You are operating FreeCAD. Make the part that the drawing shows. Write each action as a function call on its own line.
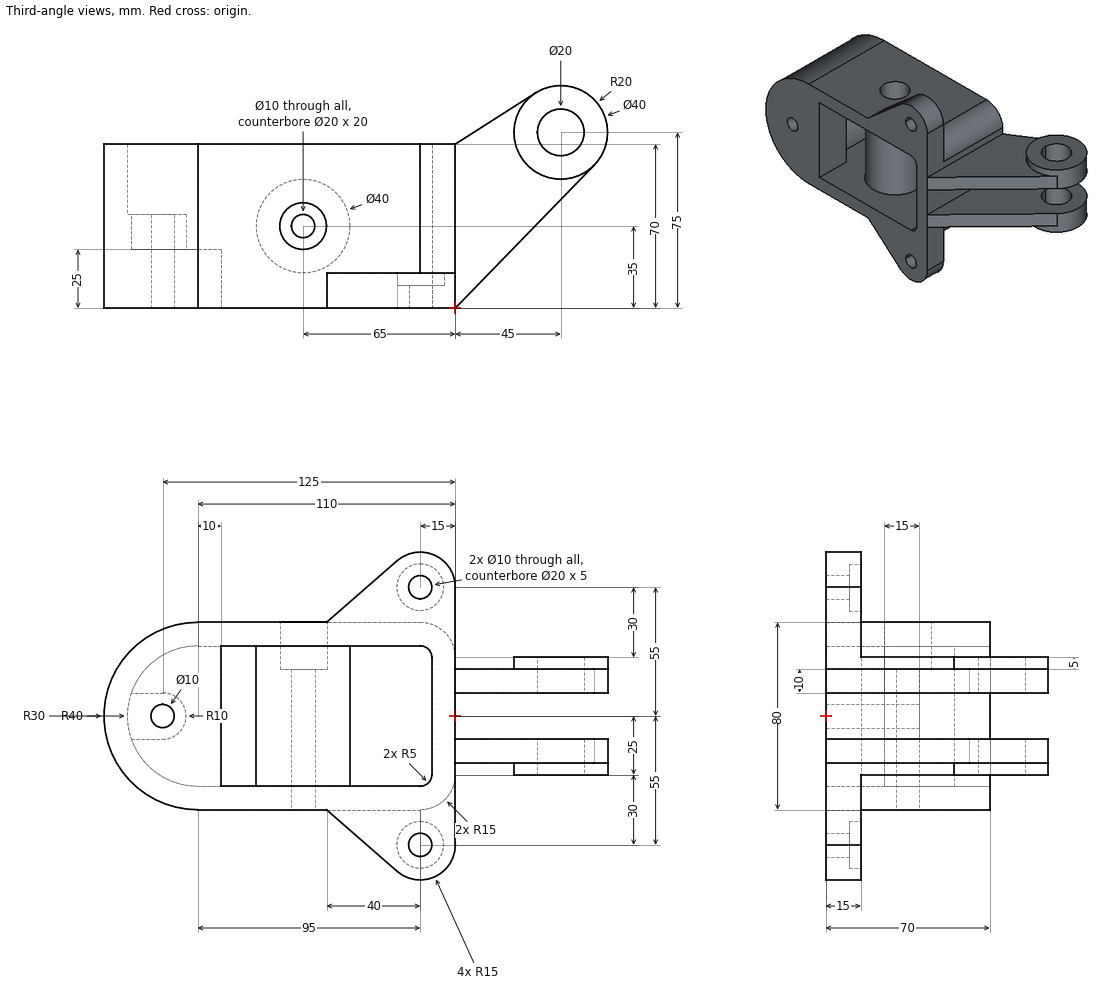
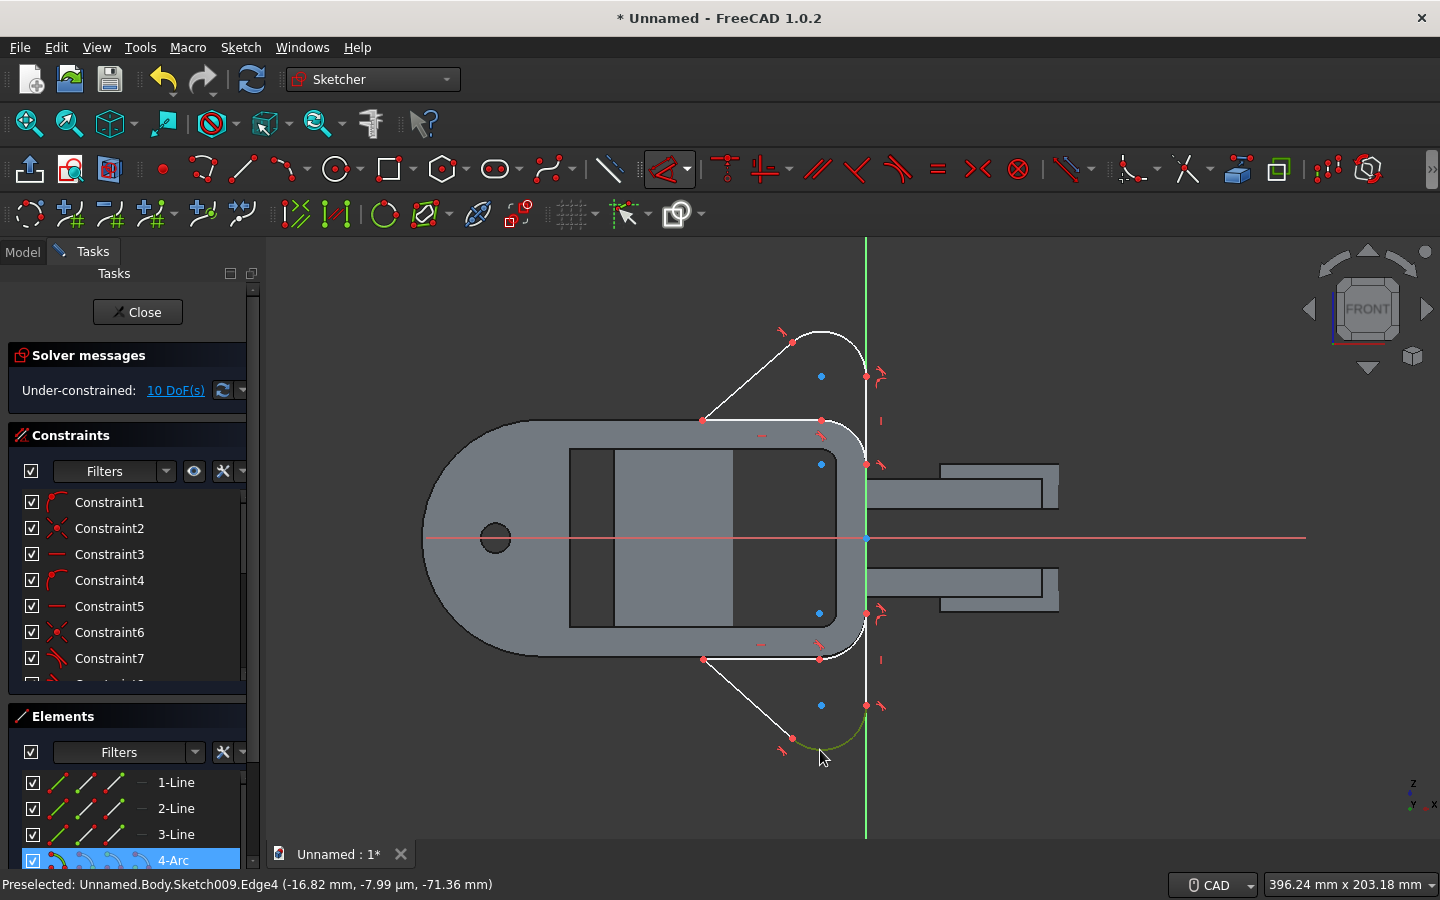
click(841, 654)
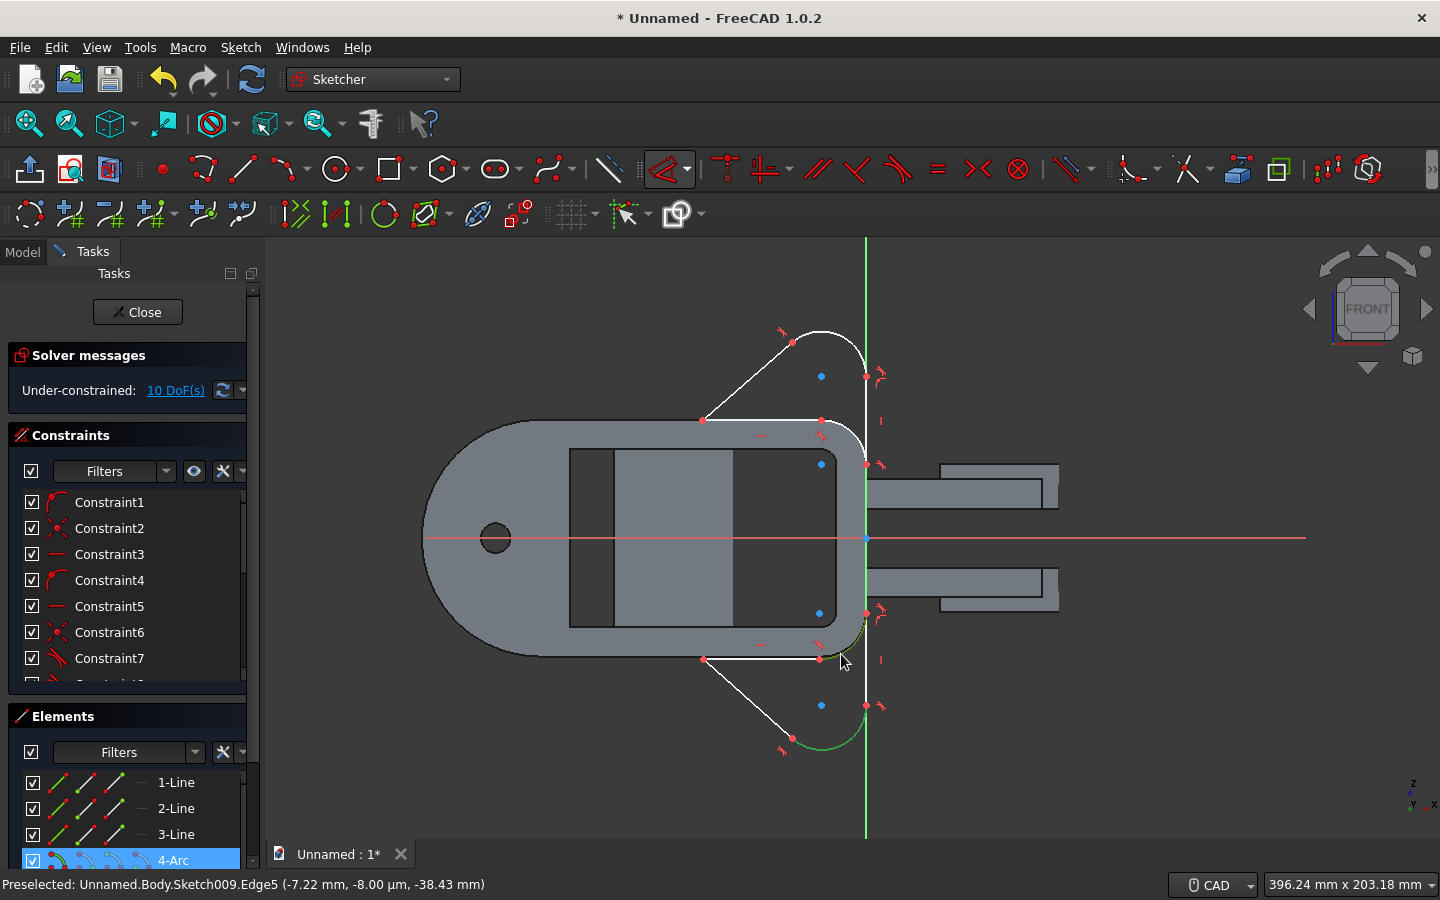
click(842, 425)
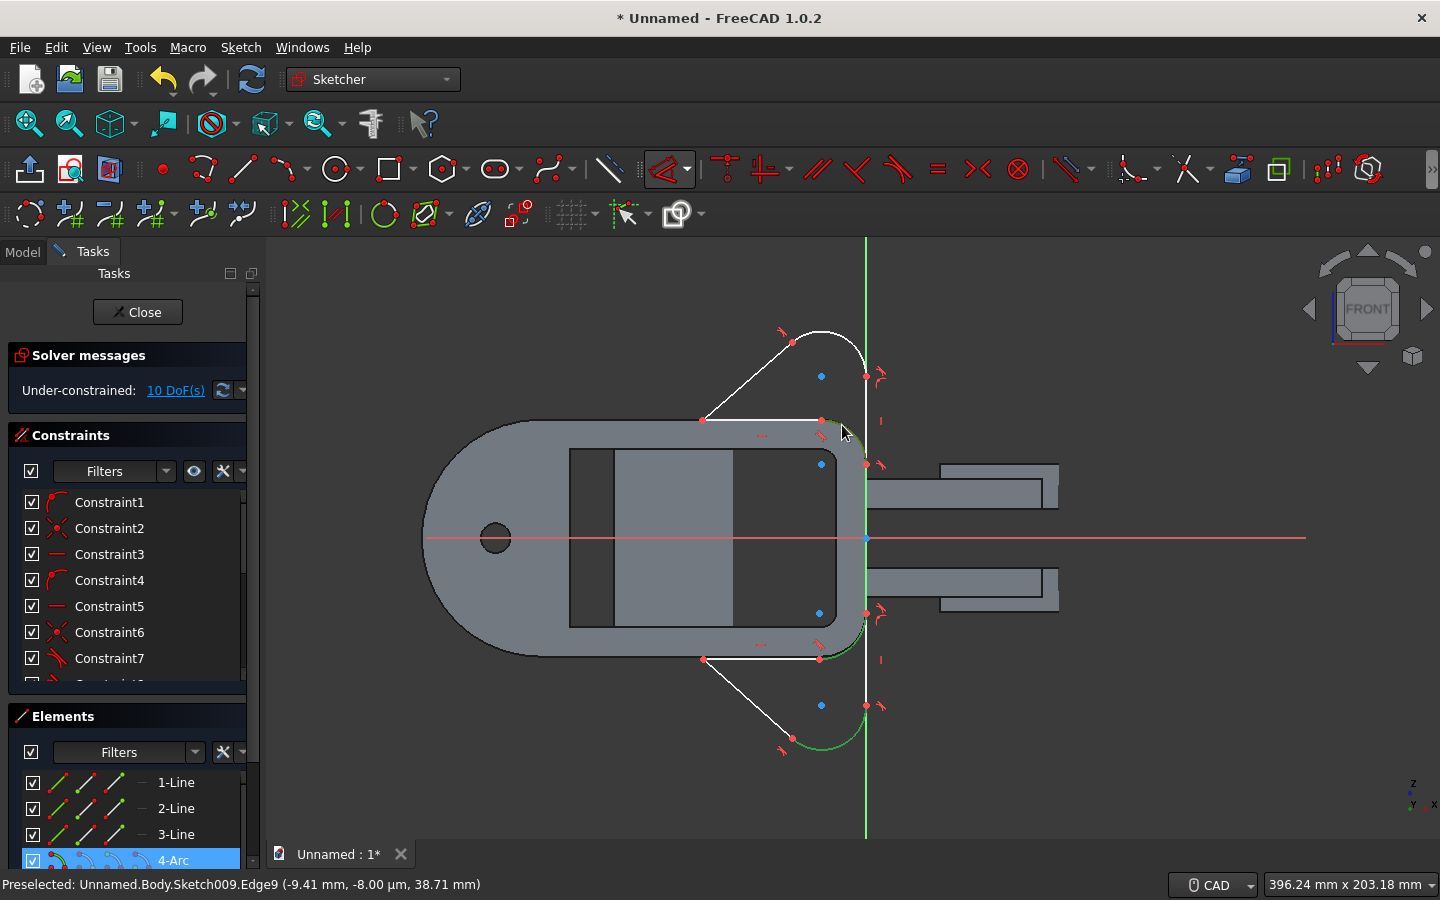
scroll(856, 348, up, 2)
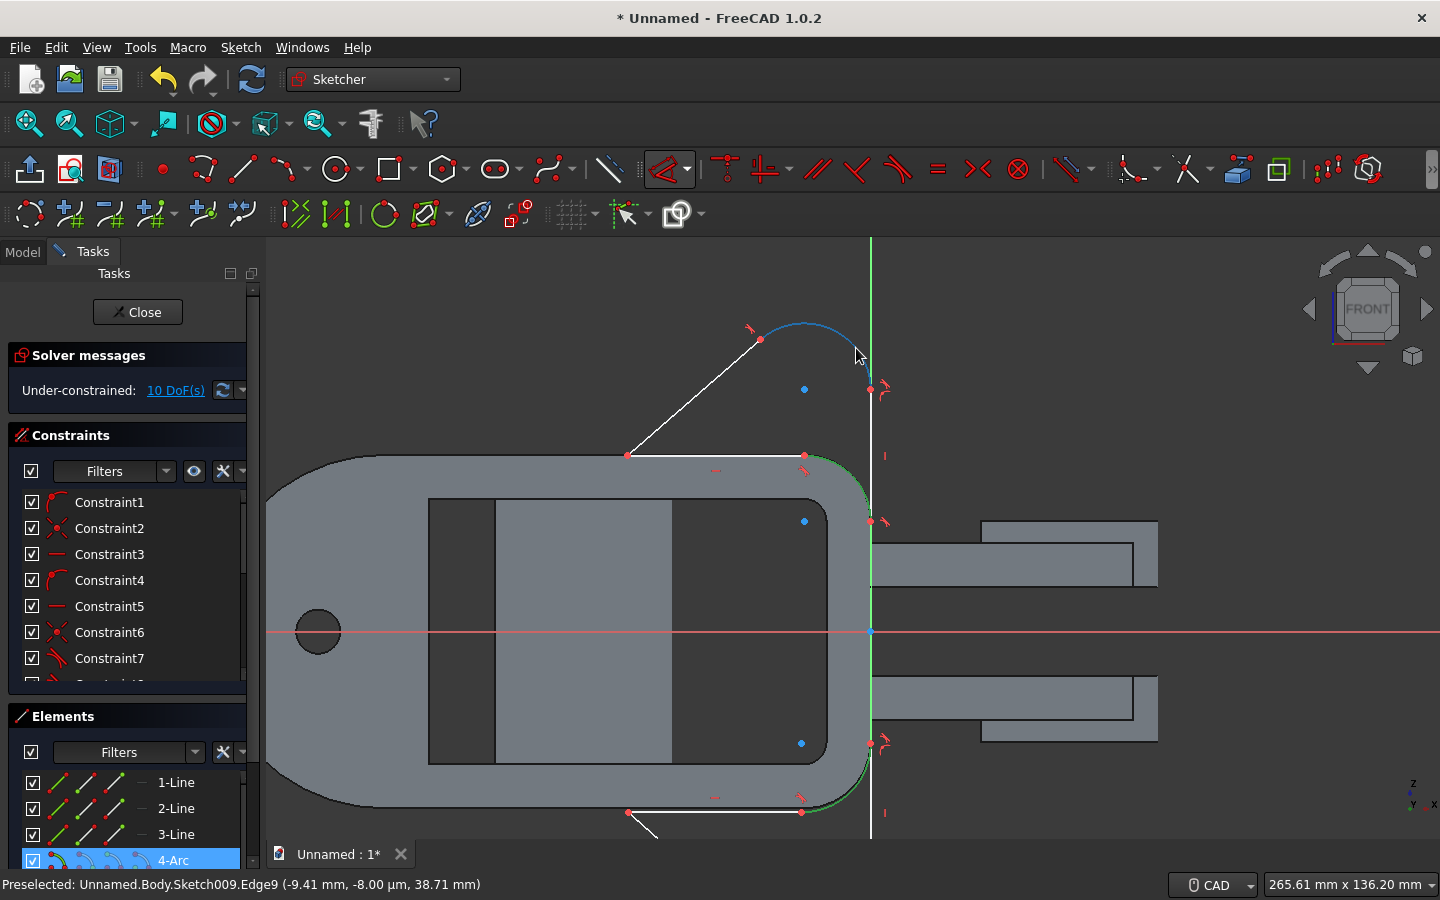
click(856, 348)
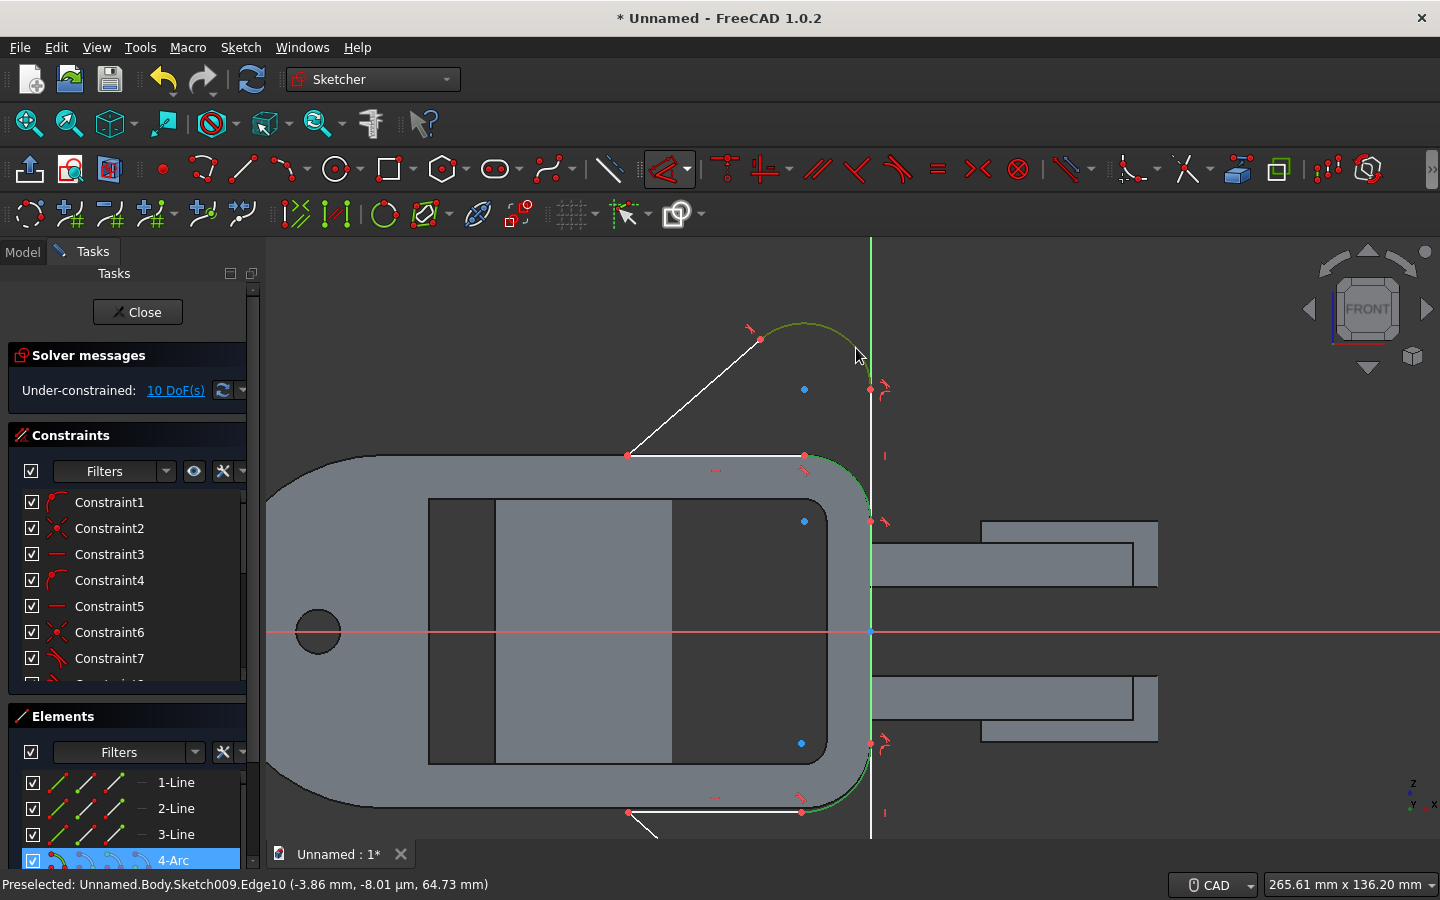
key(e)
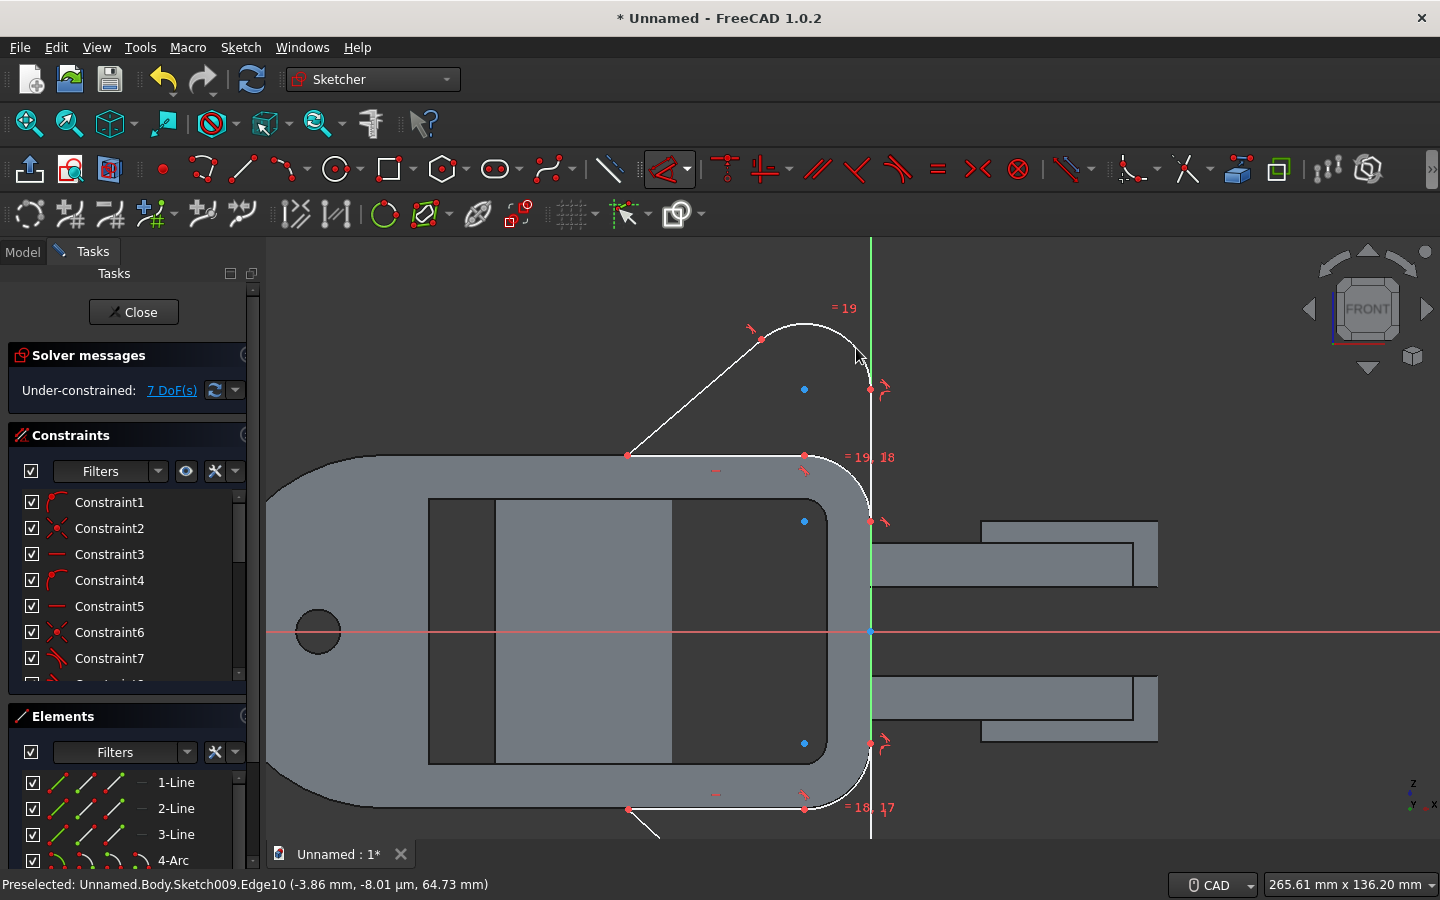
scroll(856, 348, down, 2)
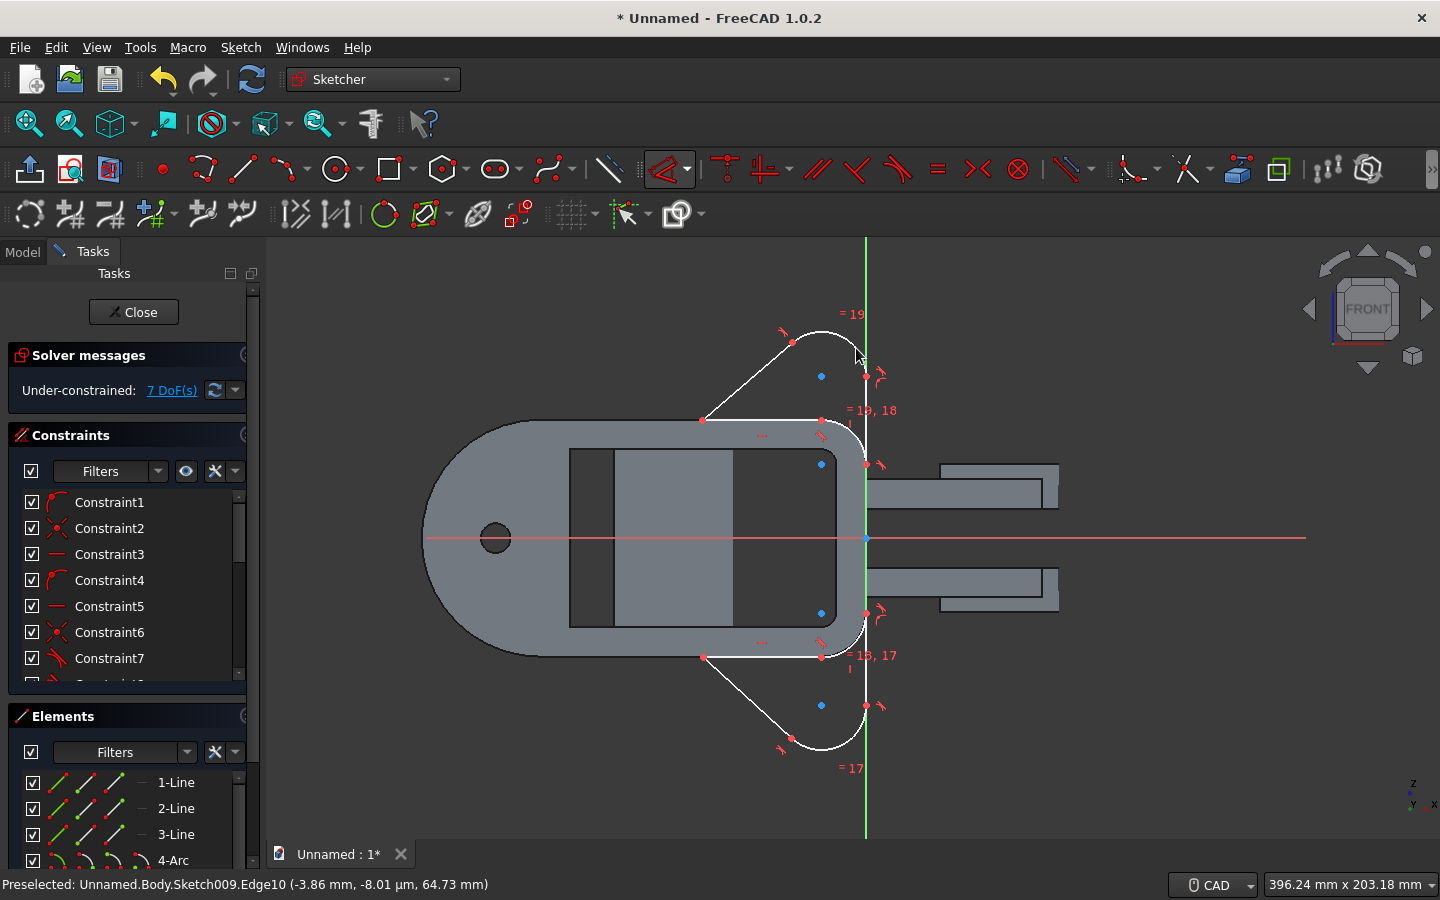
click(820, 750)